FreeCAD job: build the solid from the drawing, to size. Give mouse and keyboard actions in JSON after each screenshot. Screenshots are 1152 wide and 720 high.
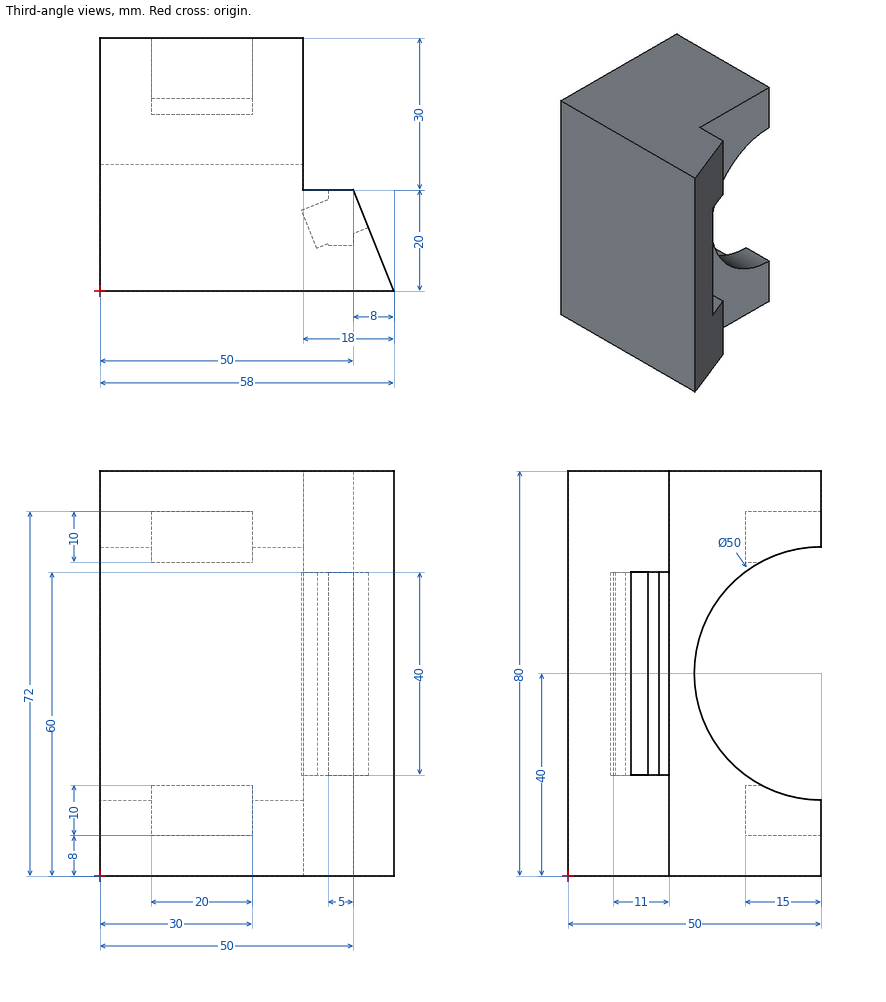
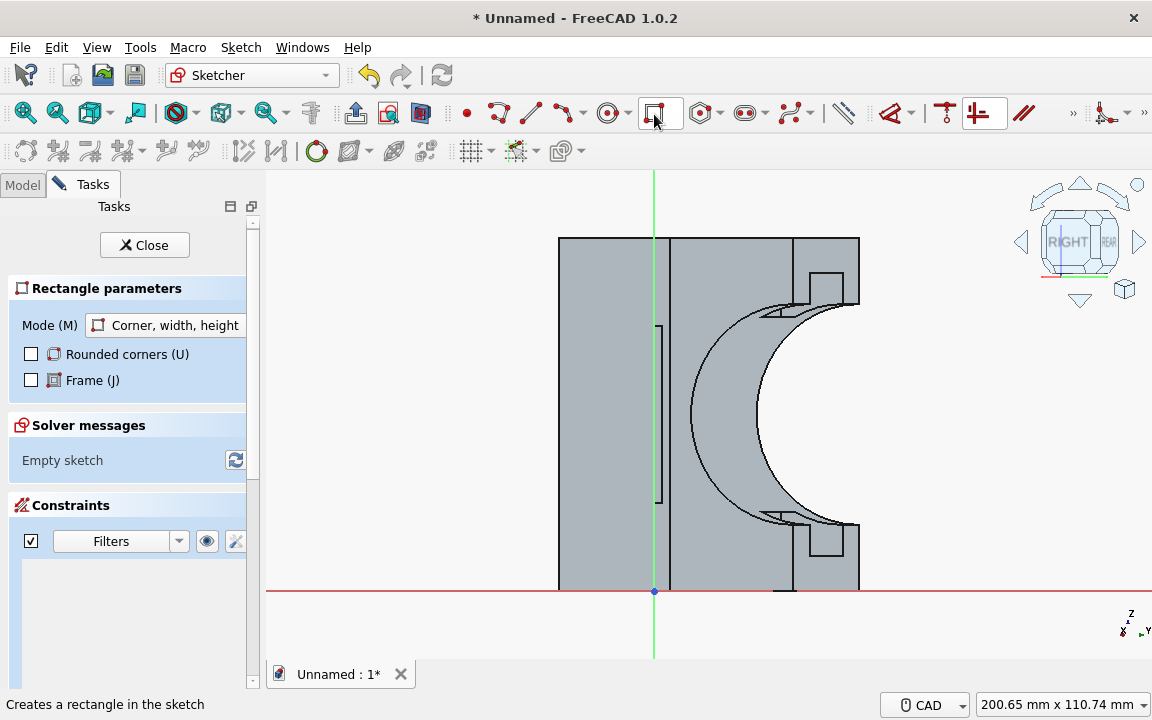
{"action": "left_click", "coordinate": [618, 326]}
{"action": "left_click", "coordinate": [654, 503]}
{"action": "key", "text": "Escape"}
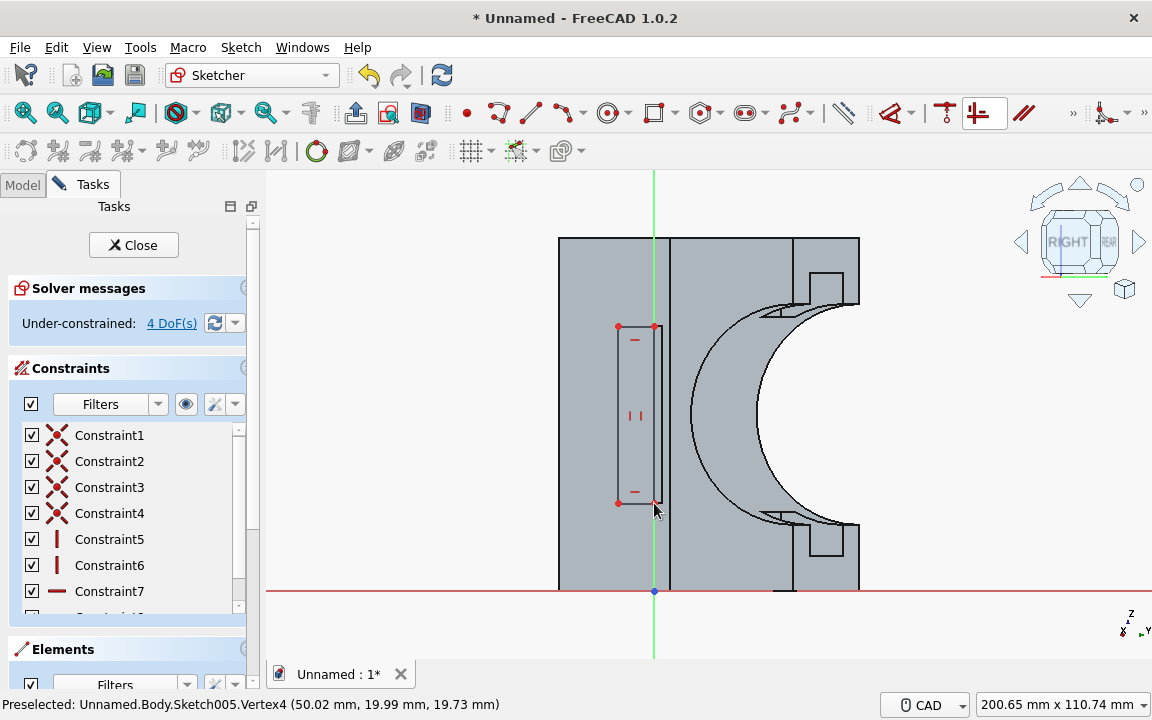
{"action": "left_click", "coordinate": [654, 504]}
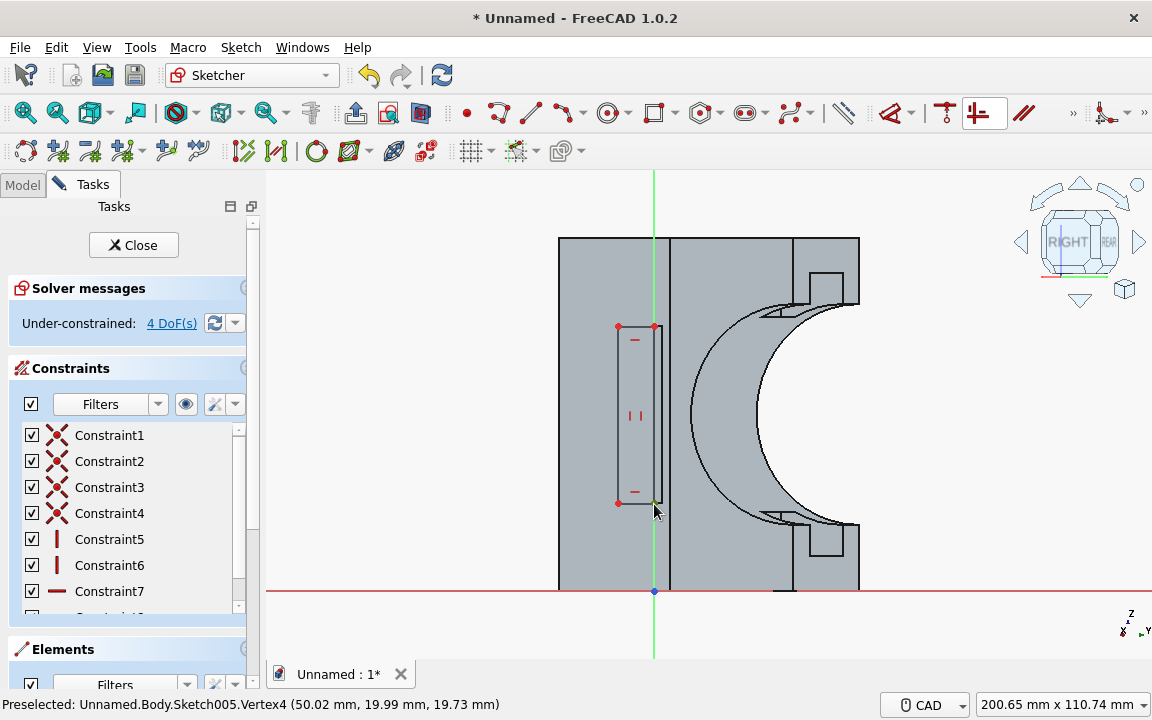
{"action": "left_click", "coordinate": [654, 538]}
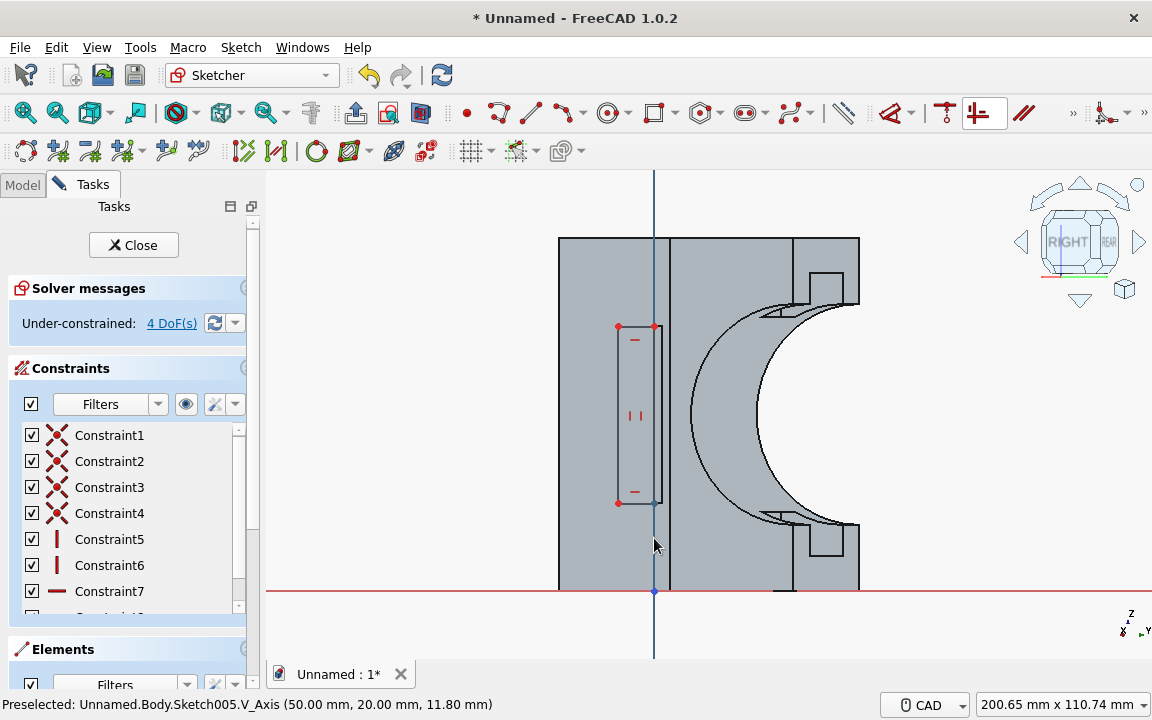
{"action": "left_click", "coordinate": [946, 114]}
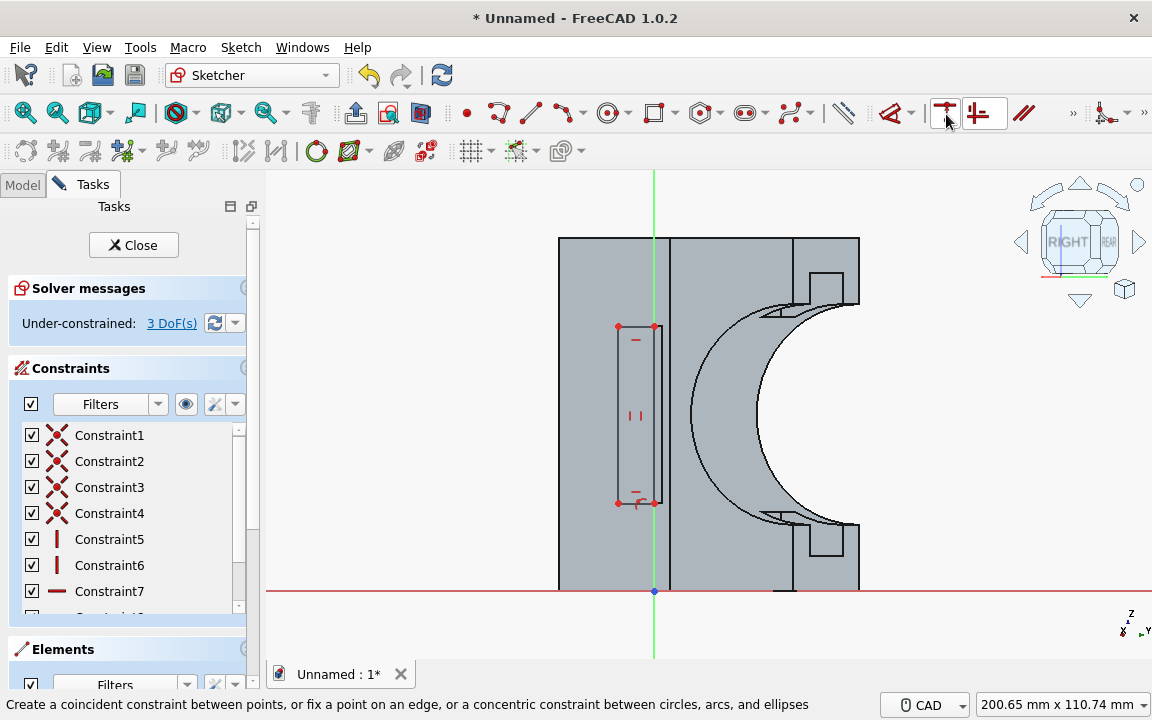
{"action": "left_click", "coordinate": [890, 114]}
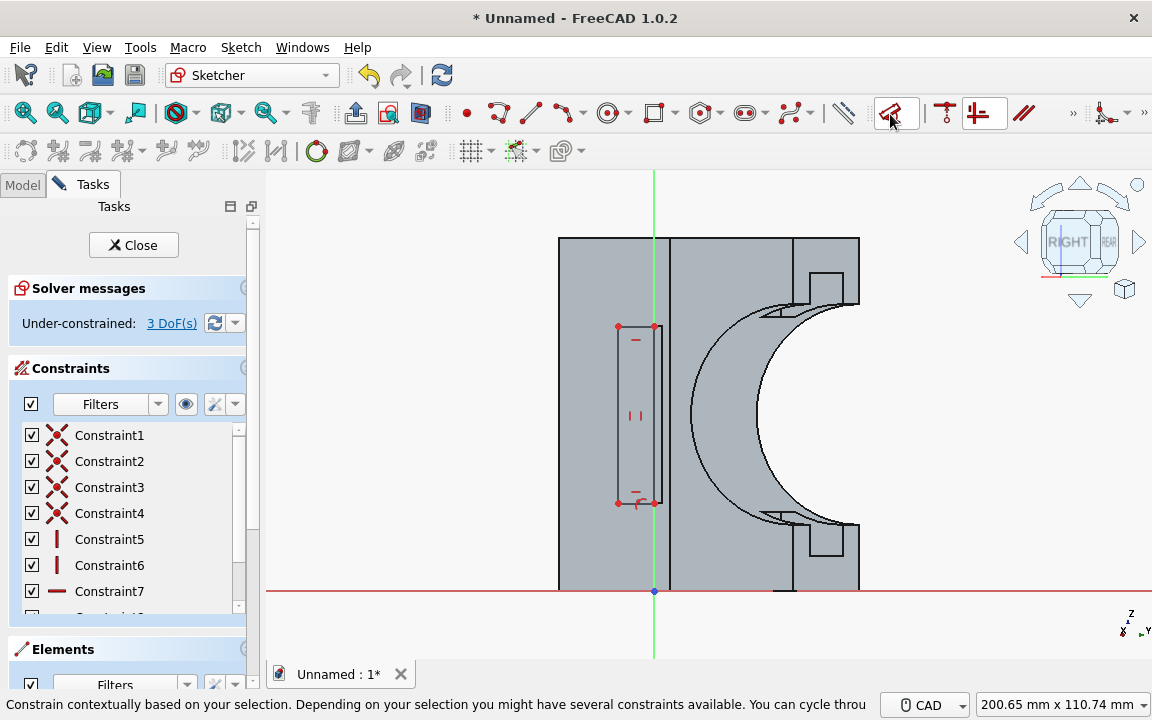
{"action": "left_click", "coordinate": [618, 380]}
{"action": "left_click", "coordinate": [584, 415]}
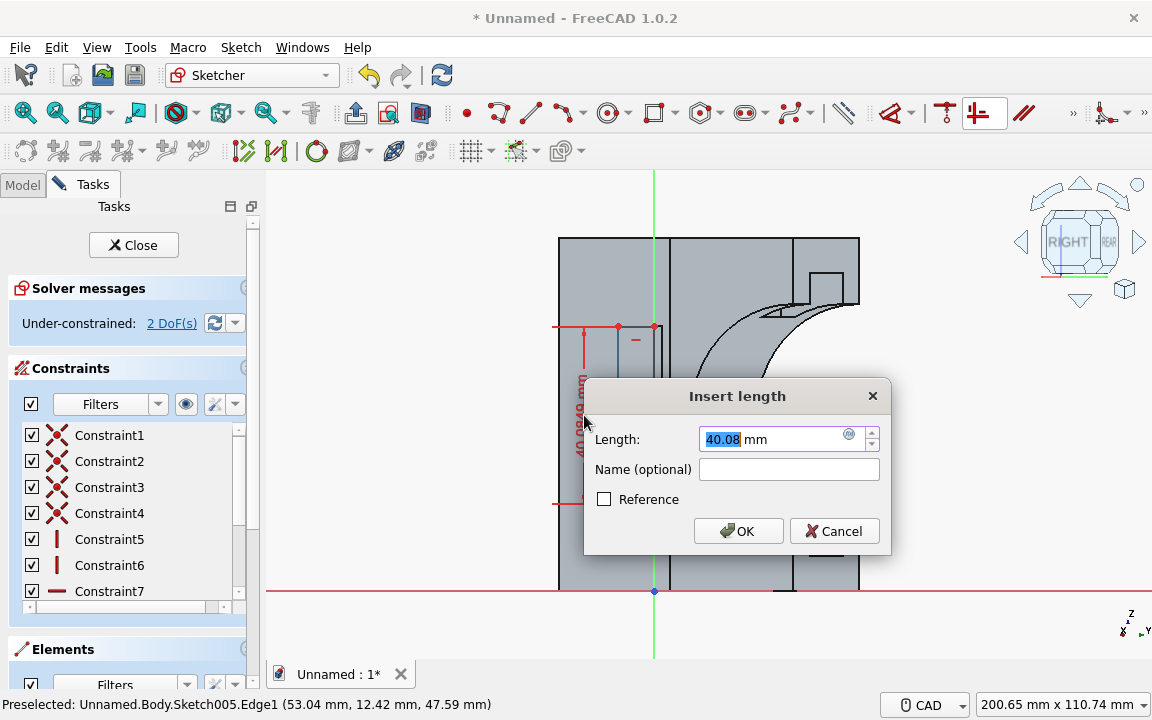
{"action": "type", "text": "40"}
{"action": "key", "text": "Return"}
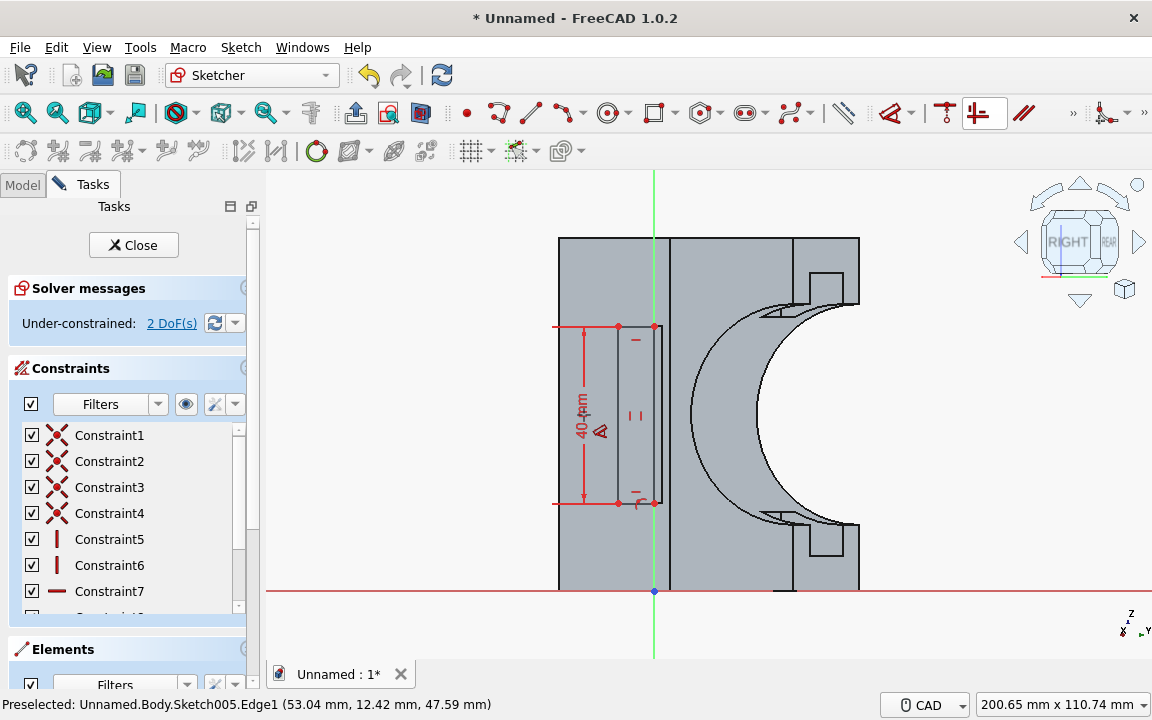
{"action": "left_click", "coordinate": [618, 327]}
{"action": "left_click", "coordinate": [584, 459]}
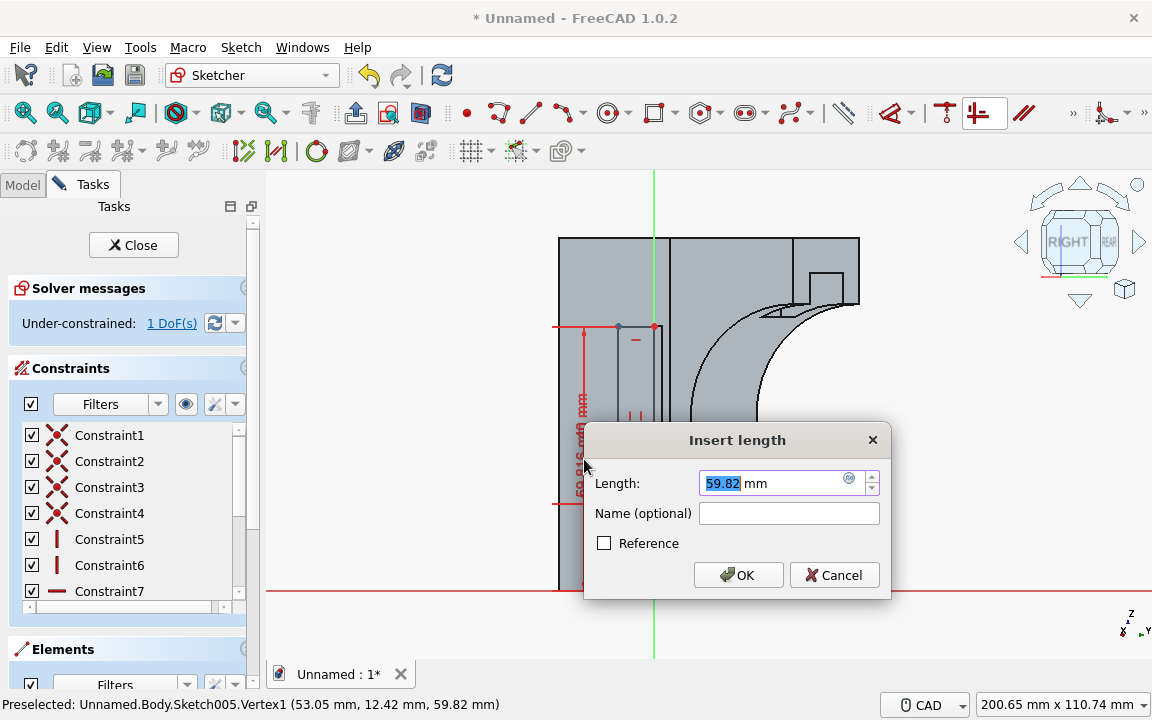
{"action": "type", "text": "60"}
{"action": "key", "text": "Return"}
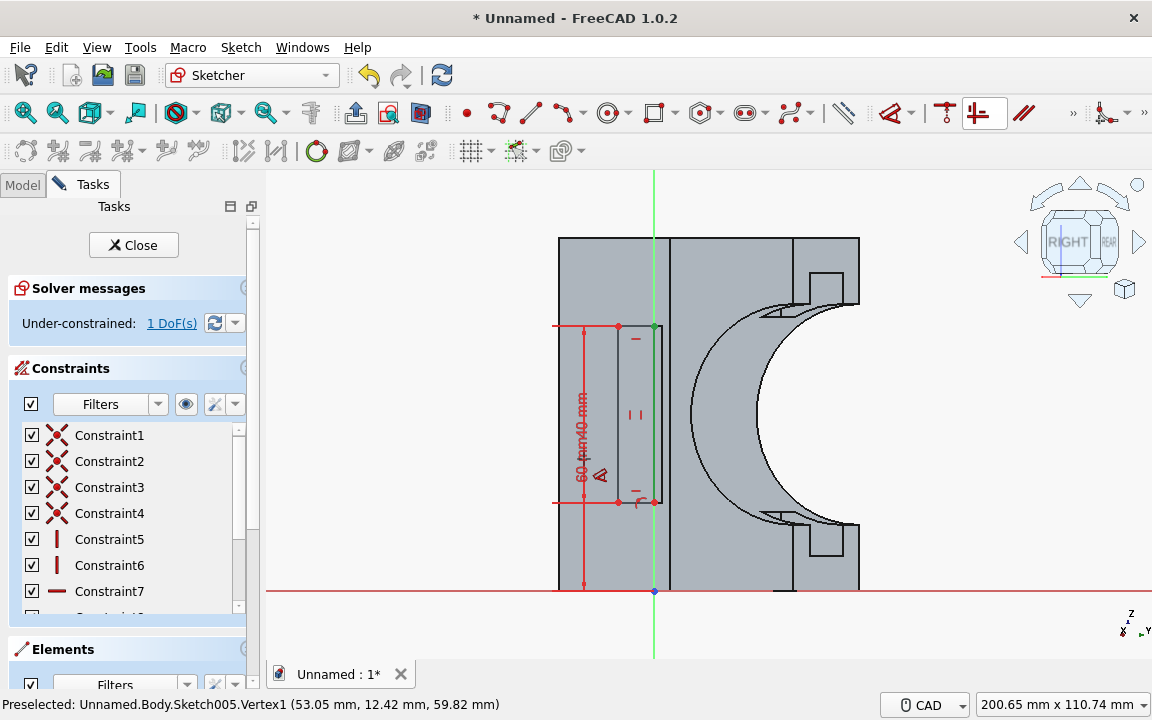
{"action": "scroll", "coordinate": [629, 503], "scroll_direction": "up", "scroll_amount": 2}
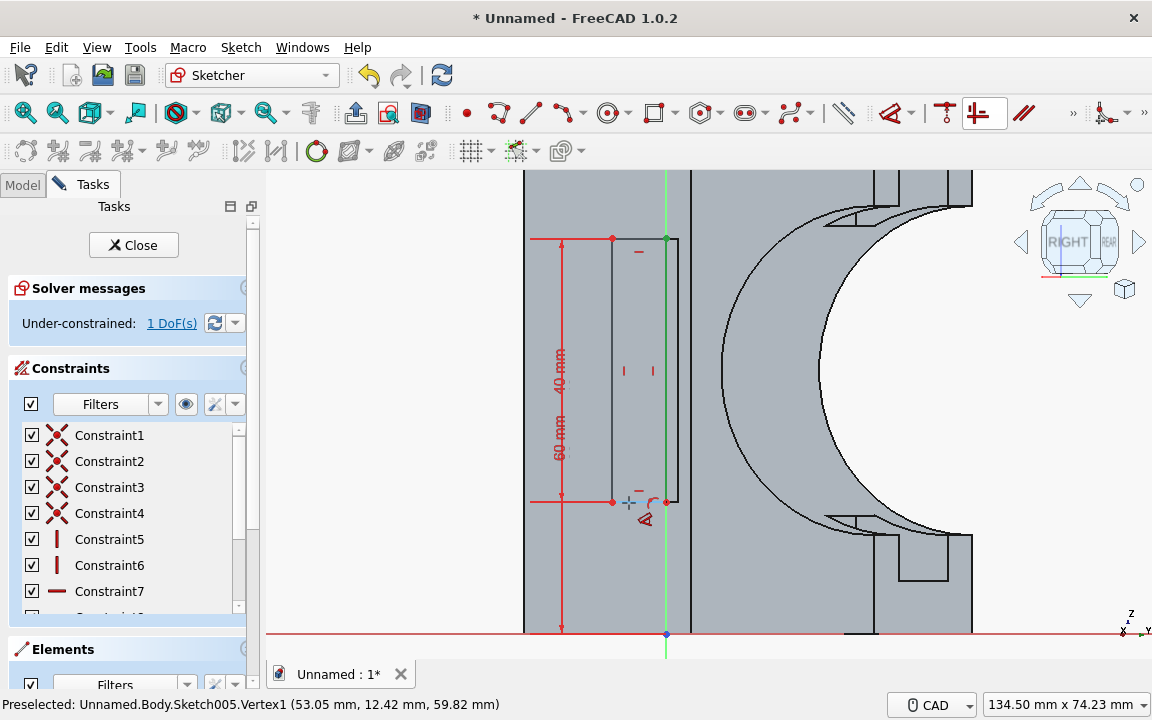
{"action": "left_click", "coordinate": [629, 502]}
{"action": "left_click", "coordinate": [639, 536]}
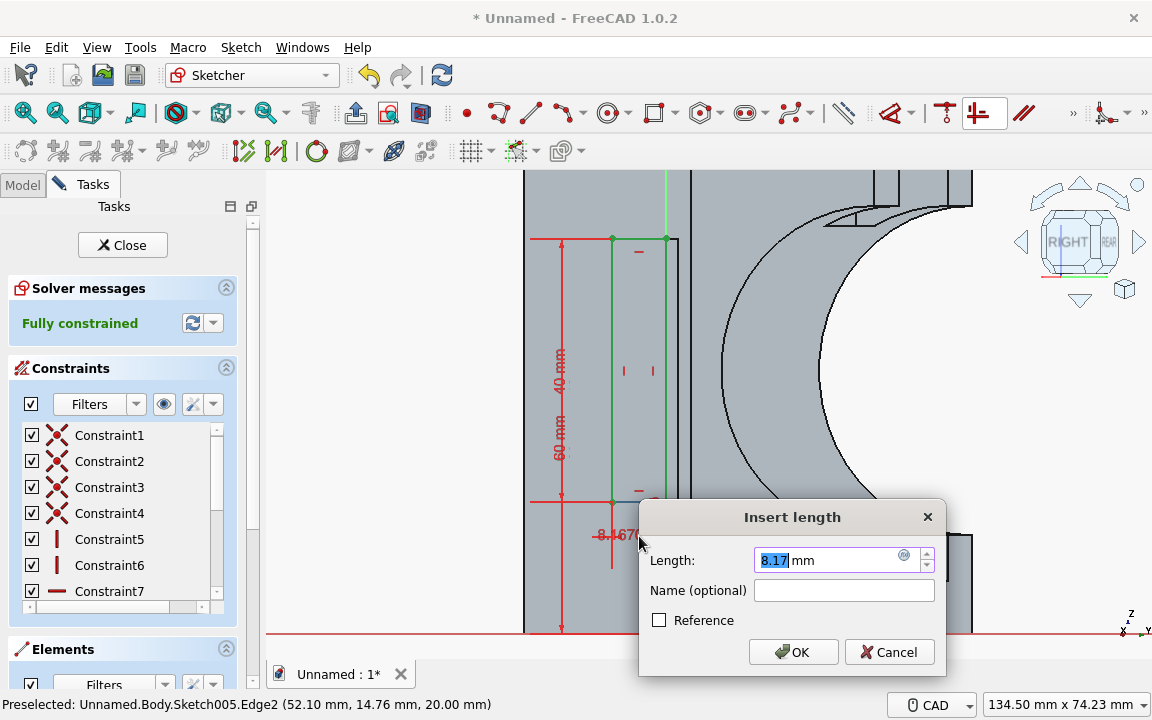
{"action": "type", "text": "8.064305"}
{"action": "key", "text": "Return"}
{"action": "key", "text": "Escape"}